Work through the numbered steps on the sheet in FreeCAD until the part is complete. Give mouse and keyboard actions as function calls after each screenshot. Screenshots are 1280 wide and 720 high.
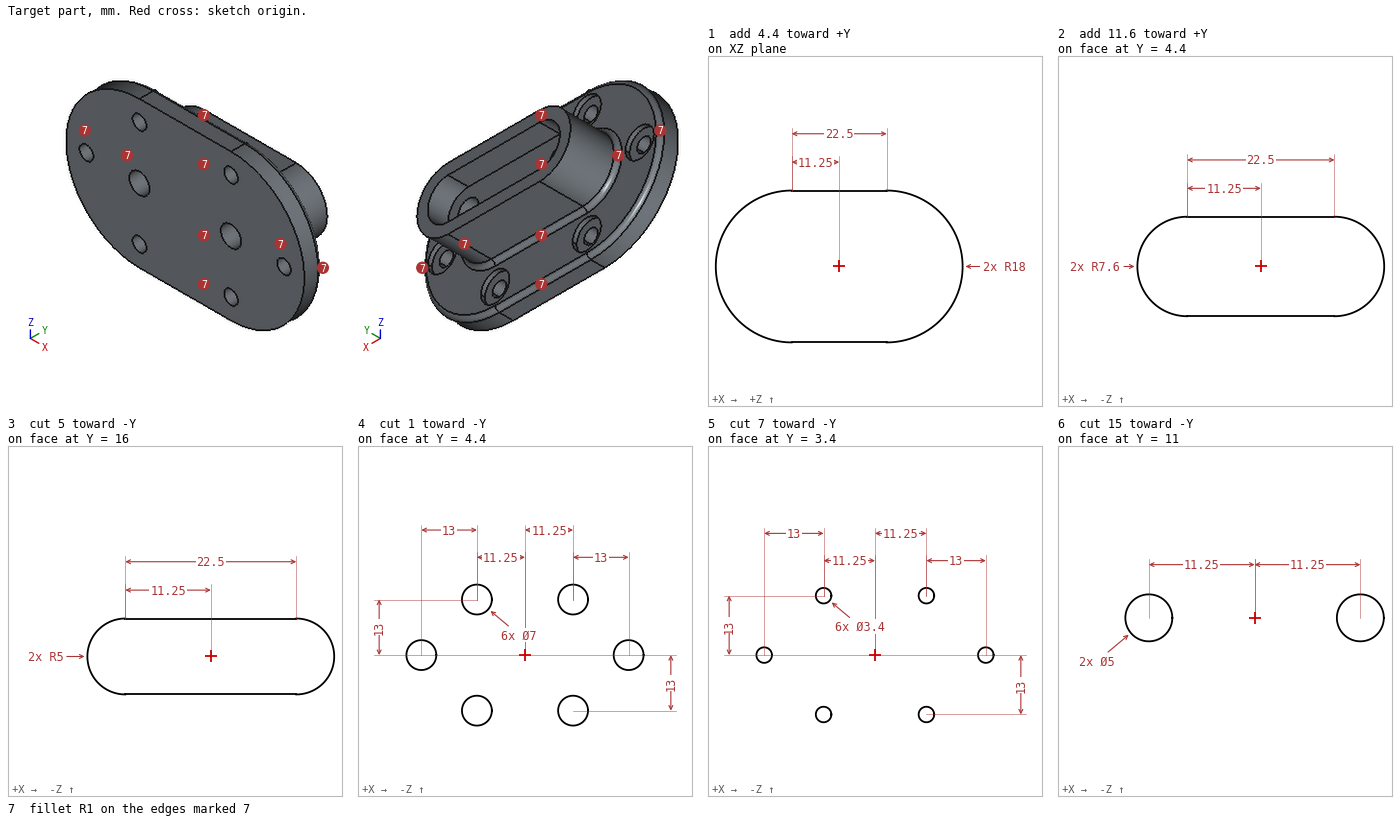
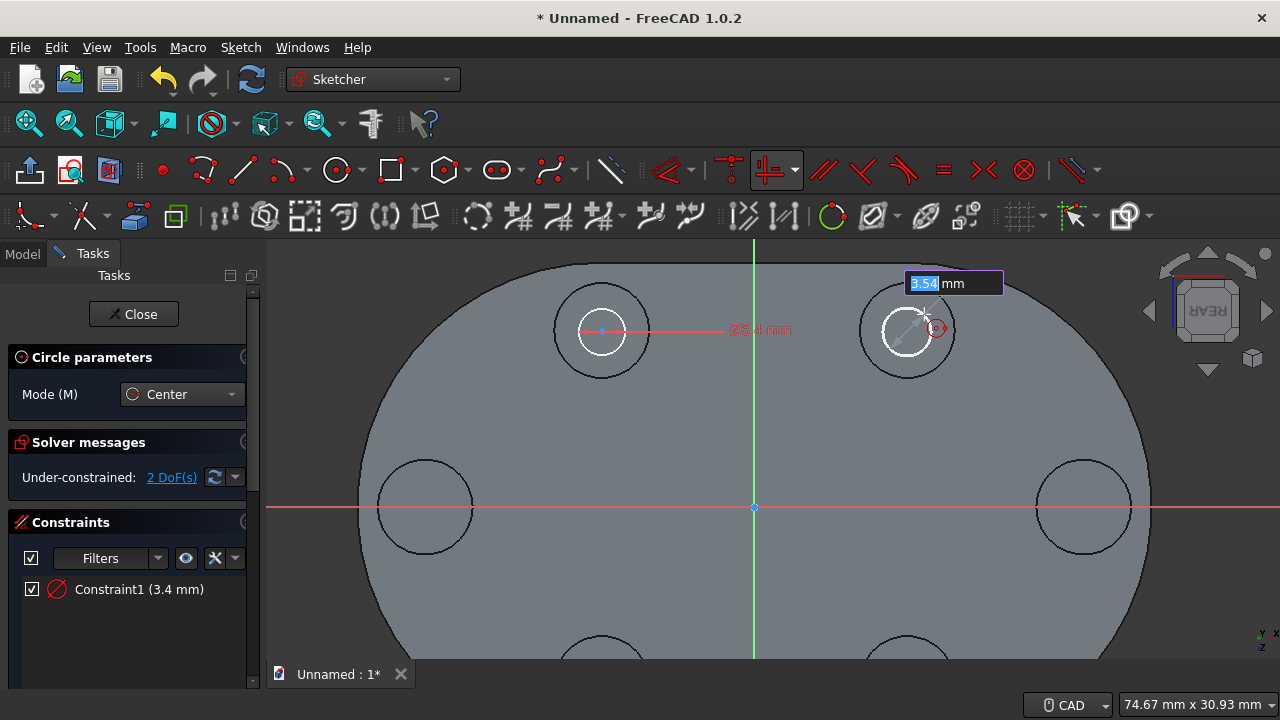
text(3.4)
key(Return)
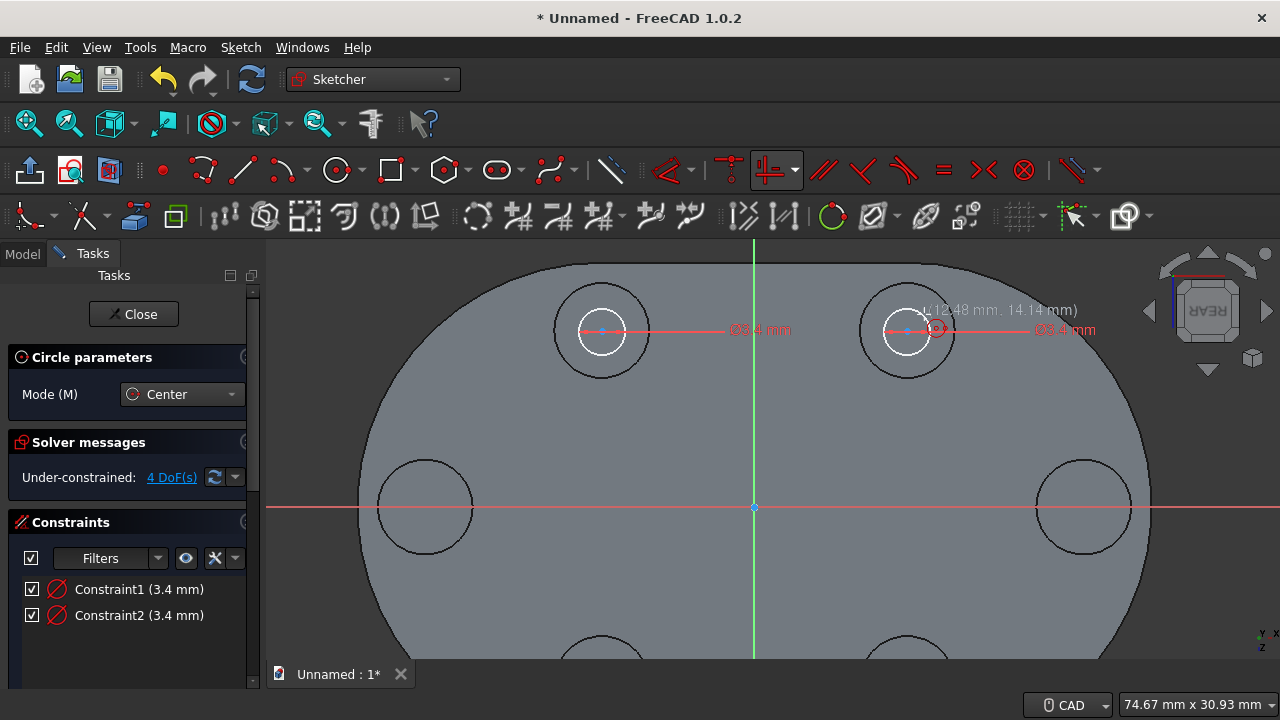
scroll(603, 331, down, 2)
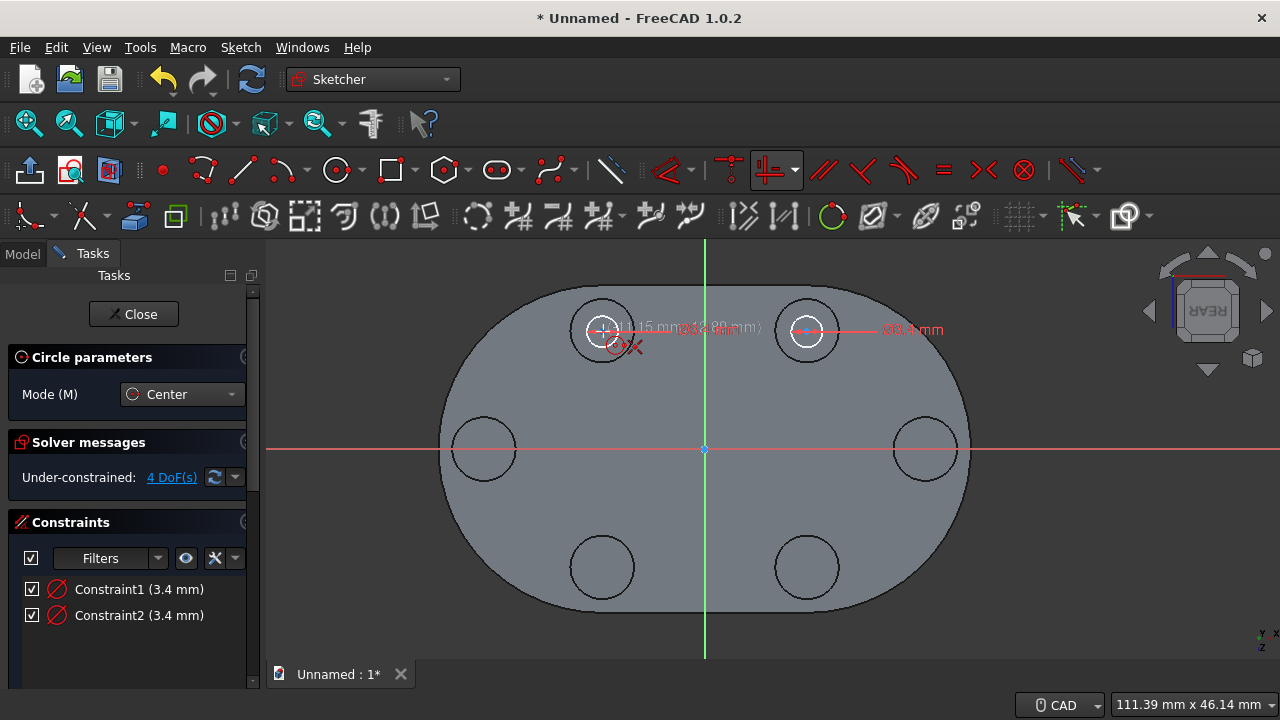
scroll(807, 567, up, 2)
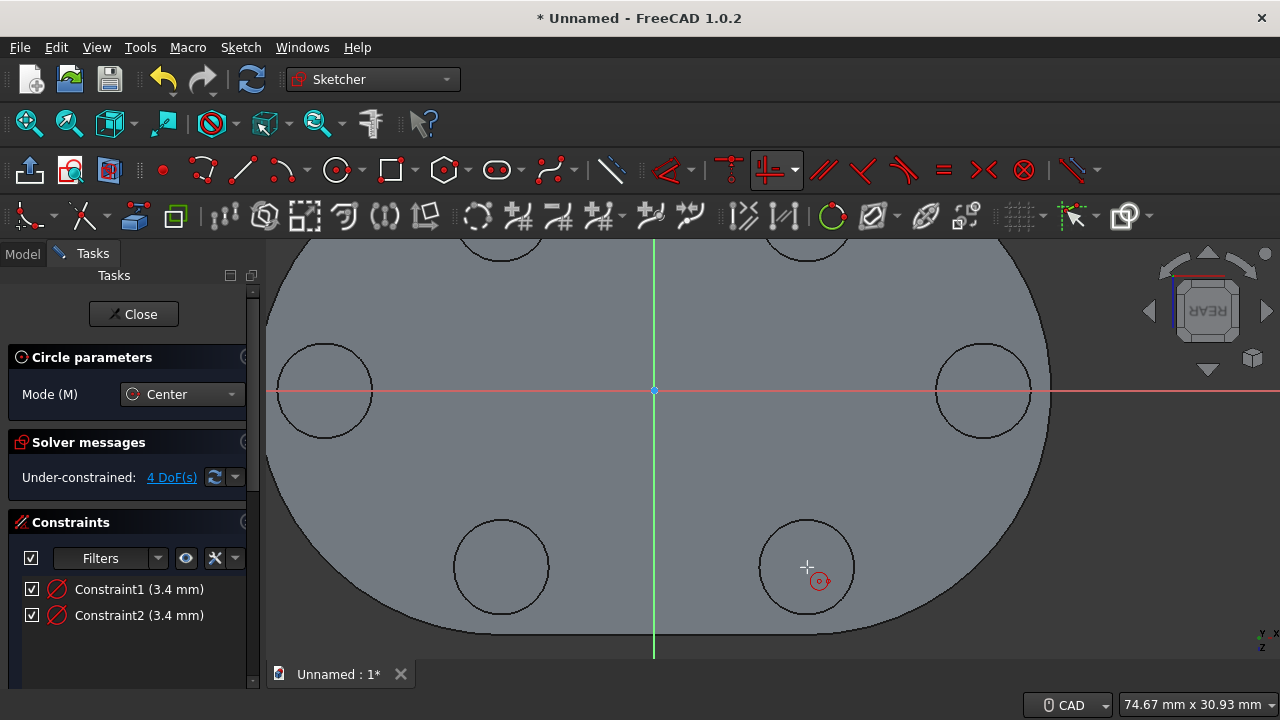
click(807, 567)
move(823, 551)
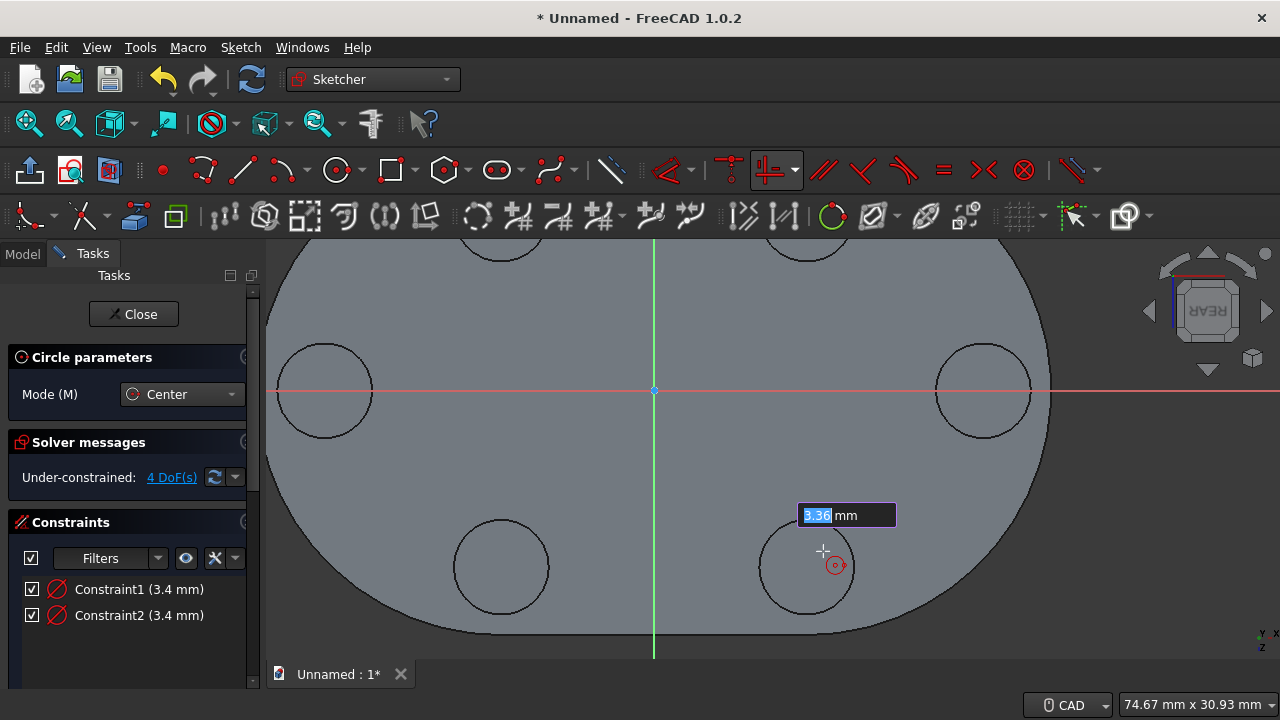
text(3.4)
key(Return)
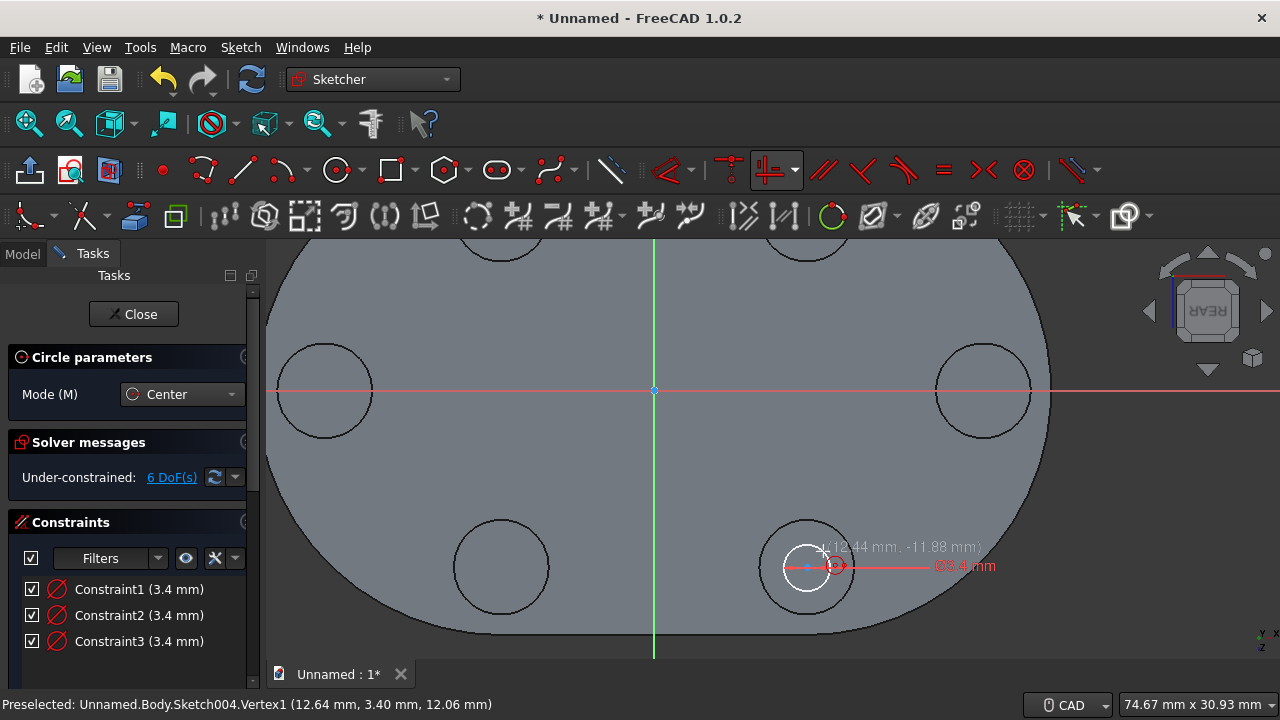
click(501, 567)
move(518, 551)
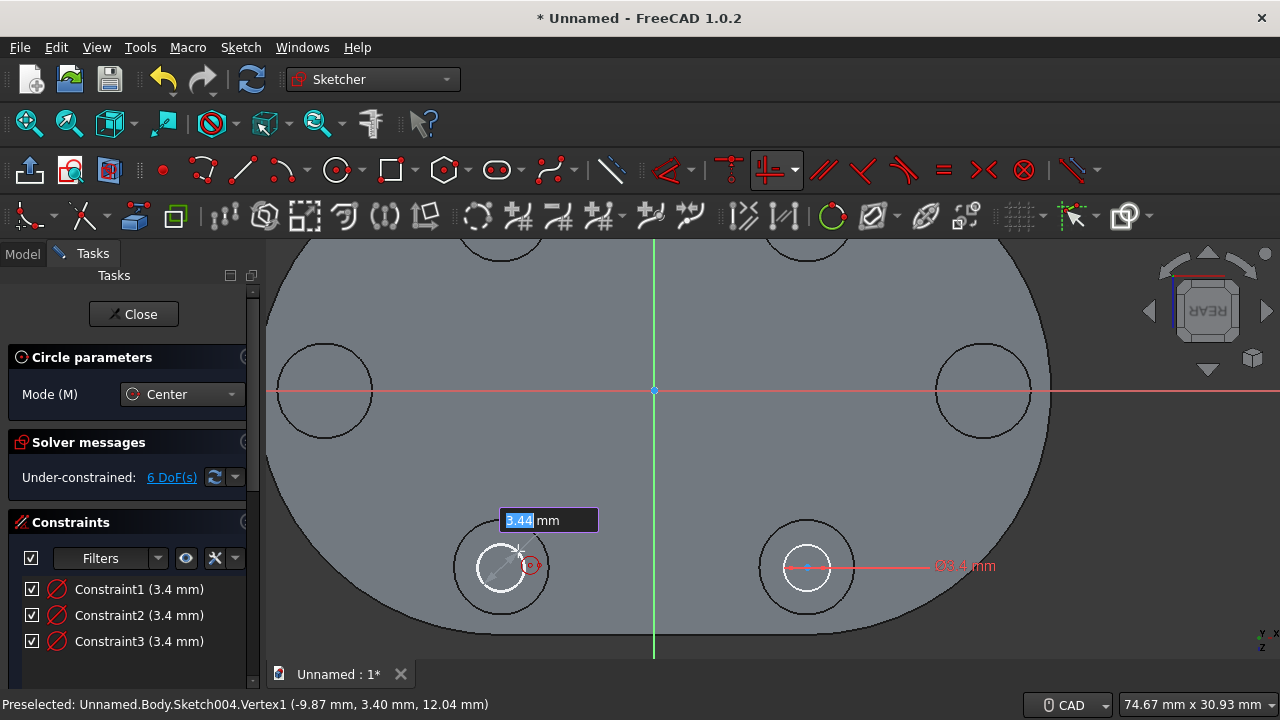
text(3.4)
key(Return)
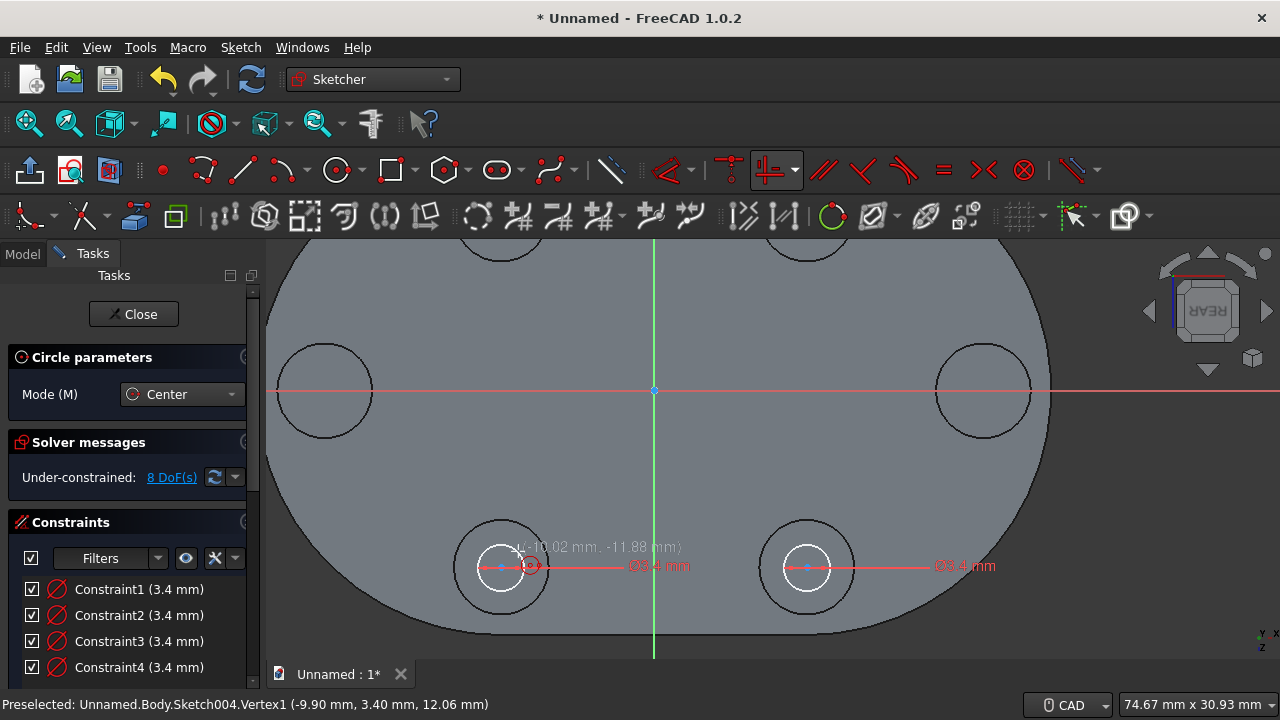
click(325, 391)
move(341, 374)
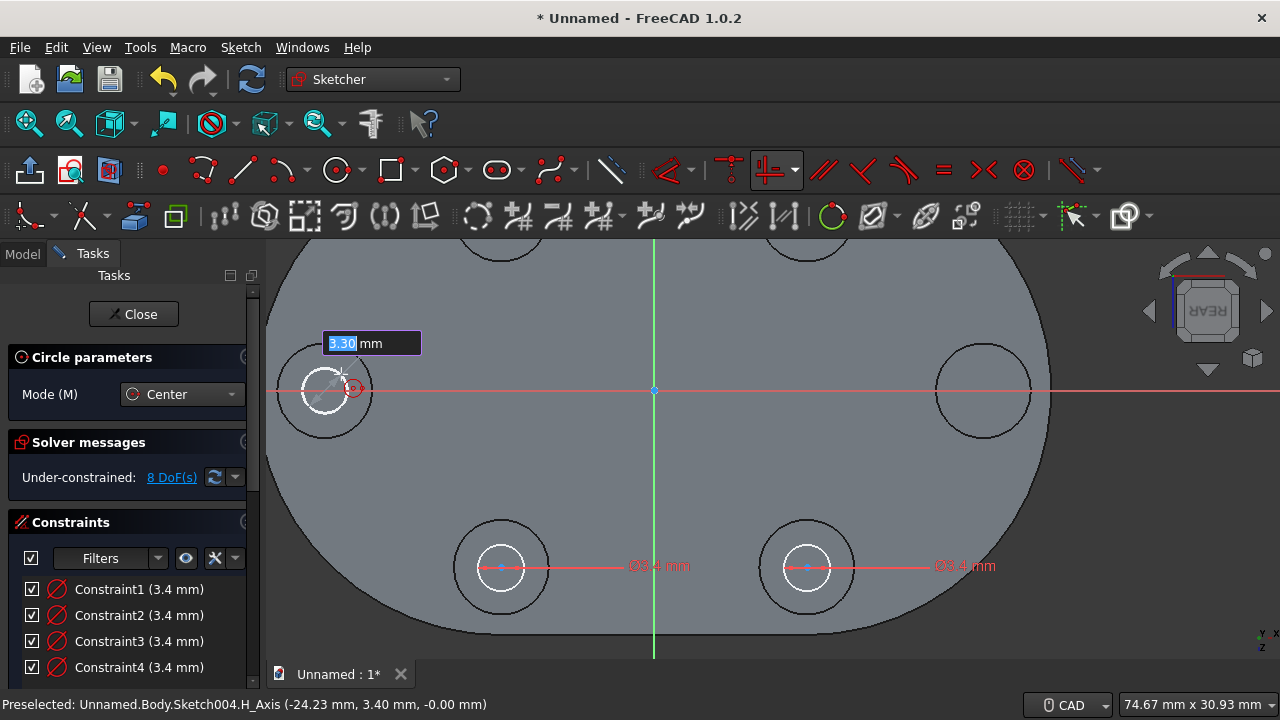
text(3.4)
key(Return)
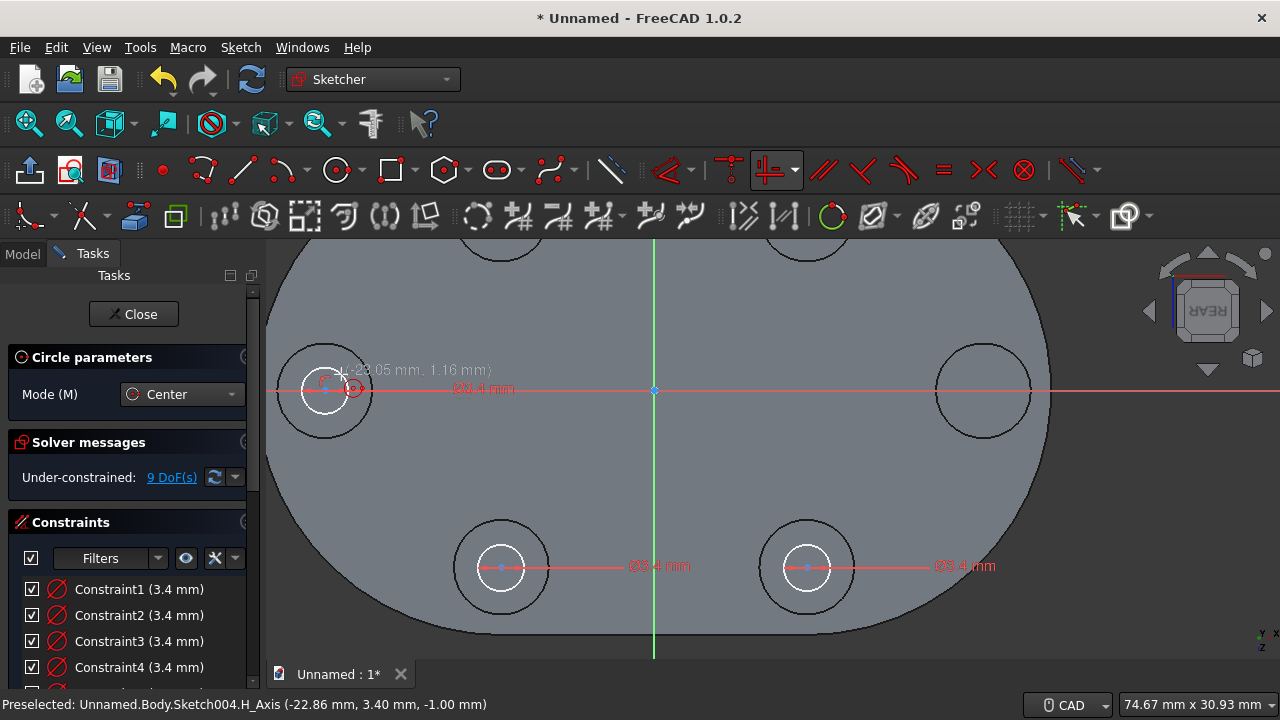
click(983, 391)
move(1000, 374)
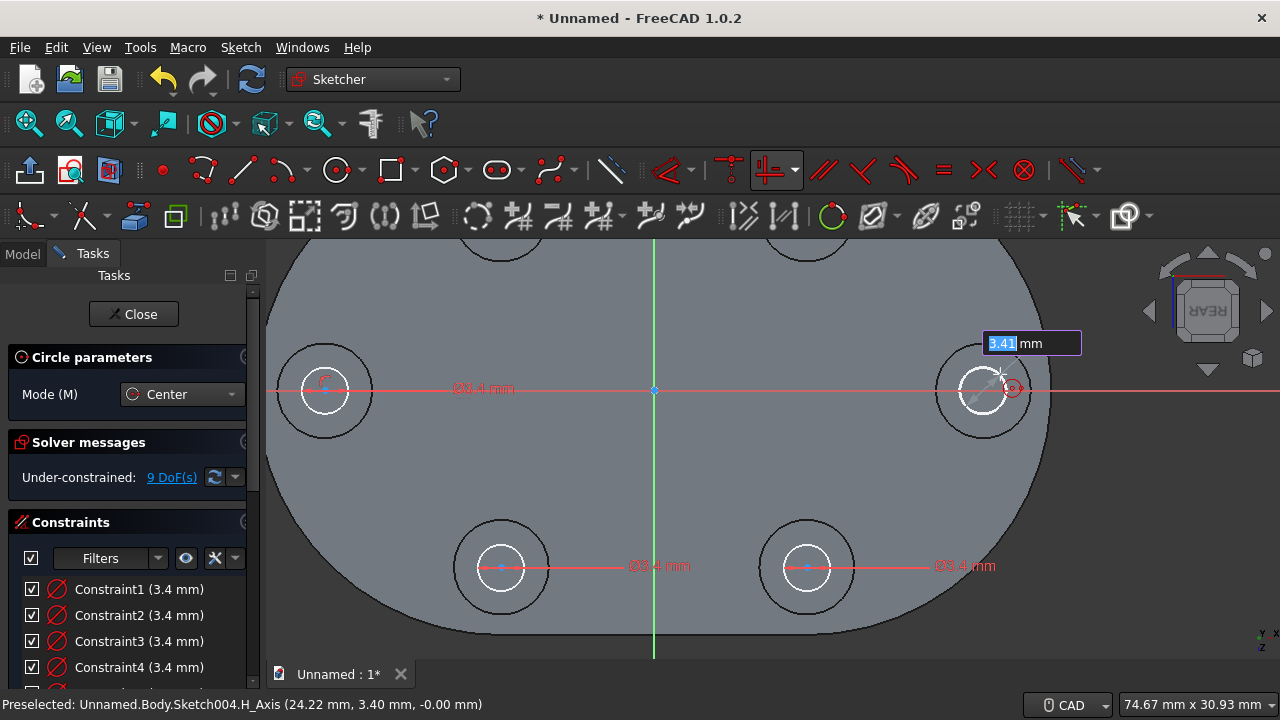
text(3.4)
key(Return)
key(Escape)